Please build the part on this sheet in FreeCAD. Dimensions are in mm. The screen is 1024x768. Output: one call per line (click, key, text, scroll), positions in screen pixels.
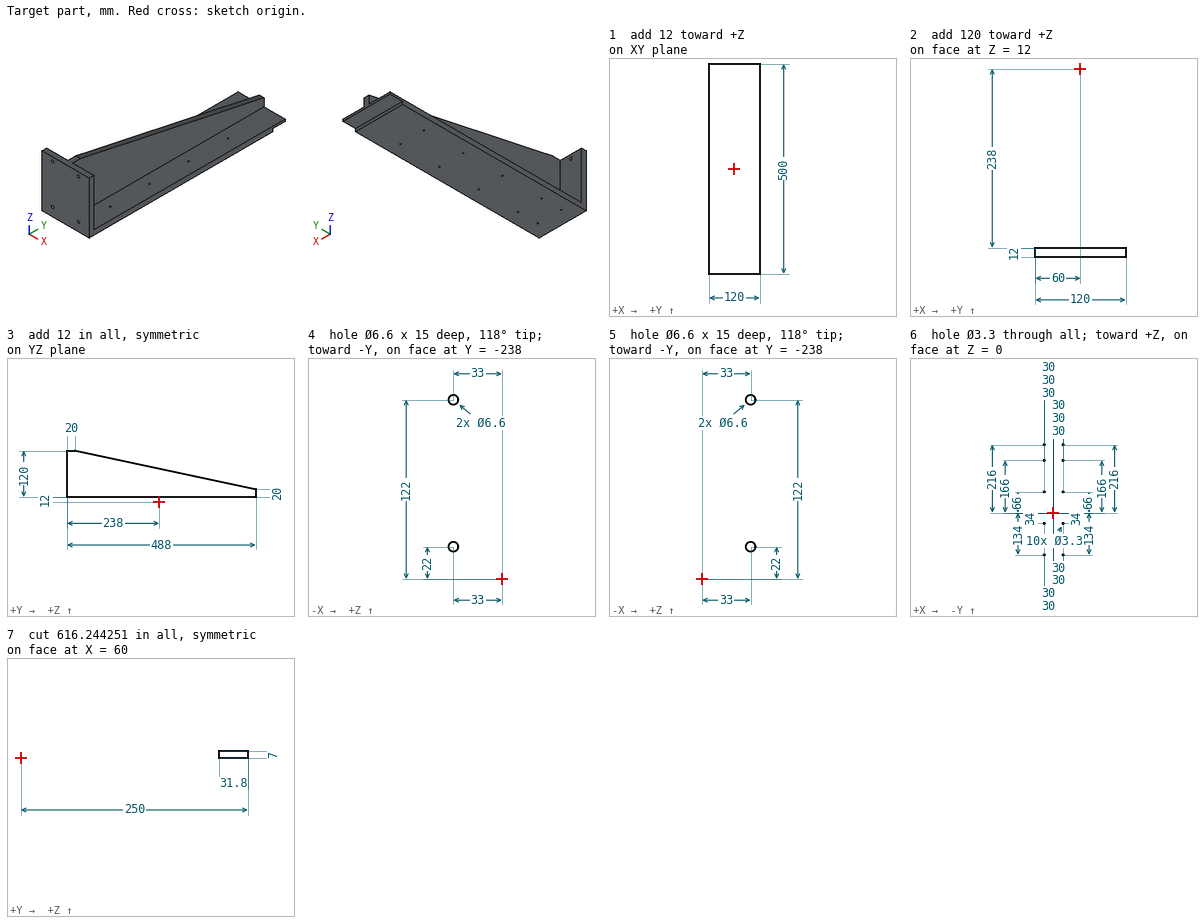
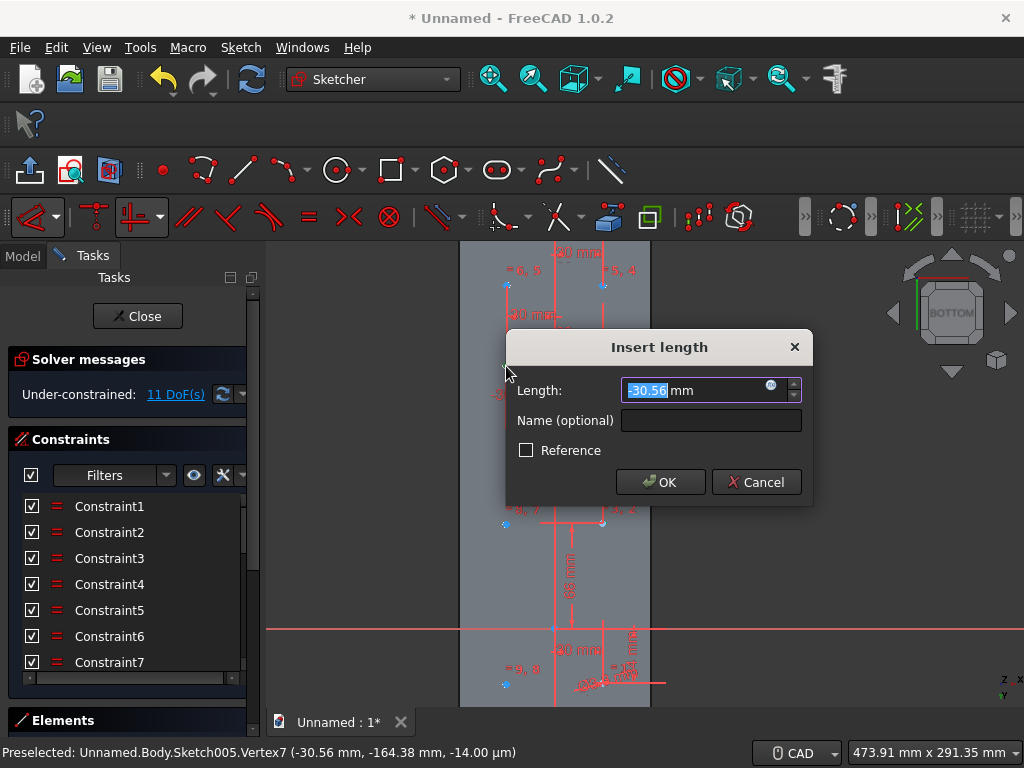
text(-30)
key(Return)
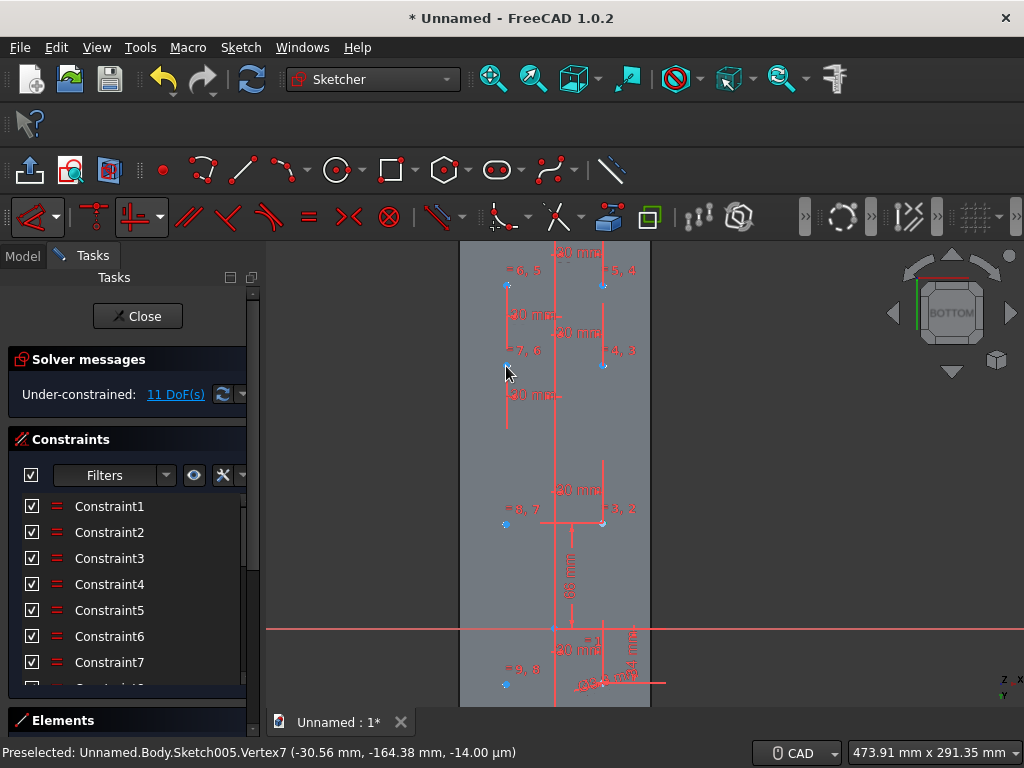
click(506, 524)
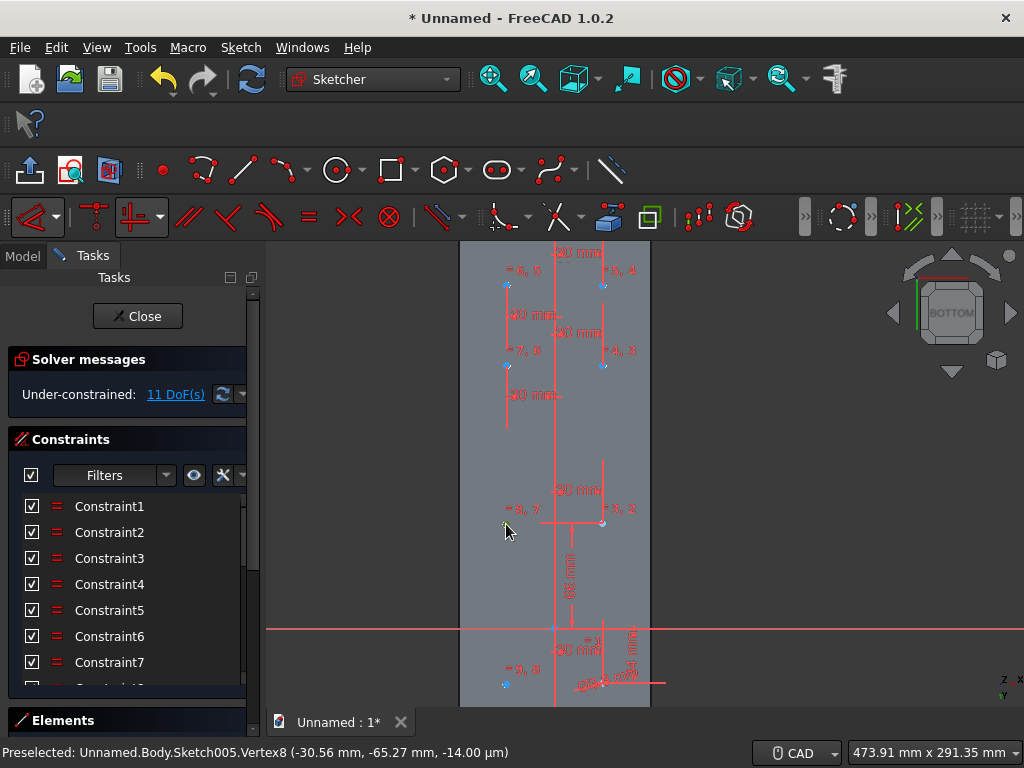
click(58, 218)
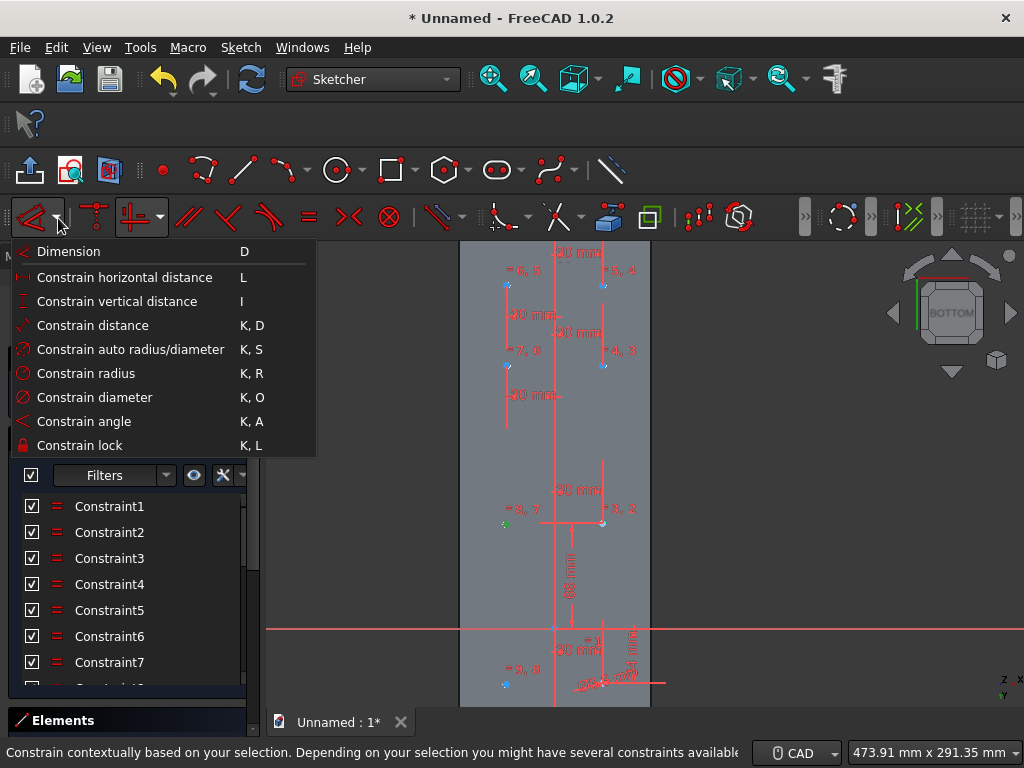
click(164, 277)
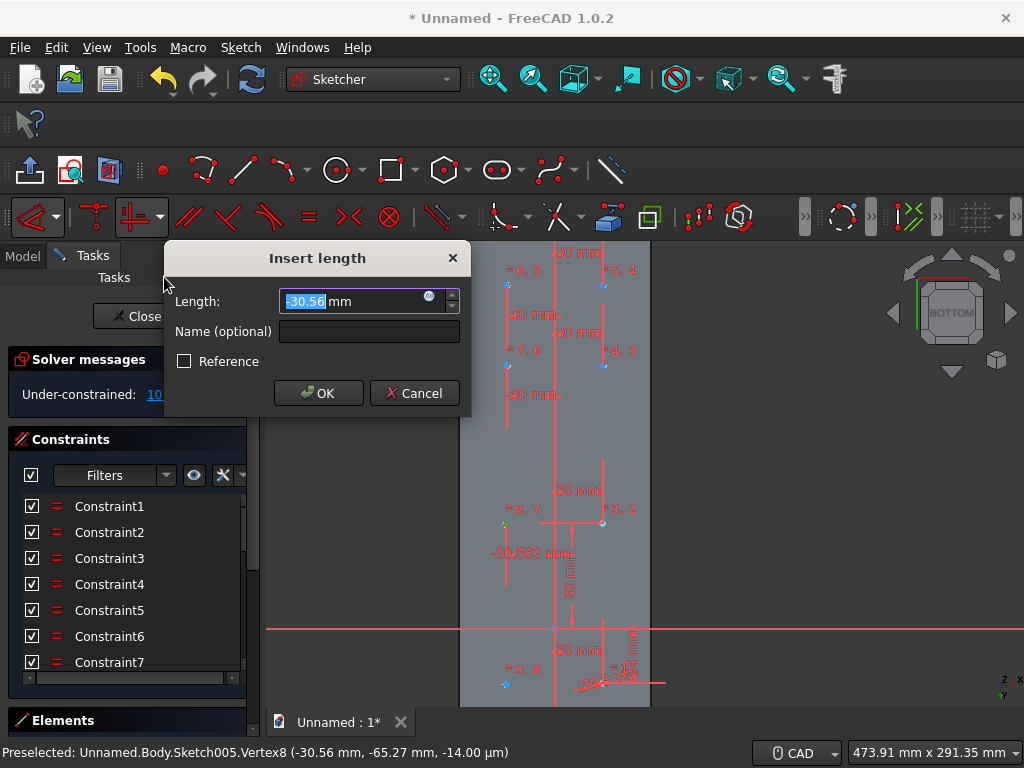
text(-30)
key(Return)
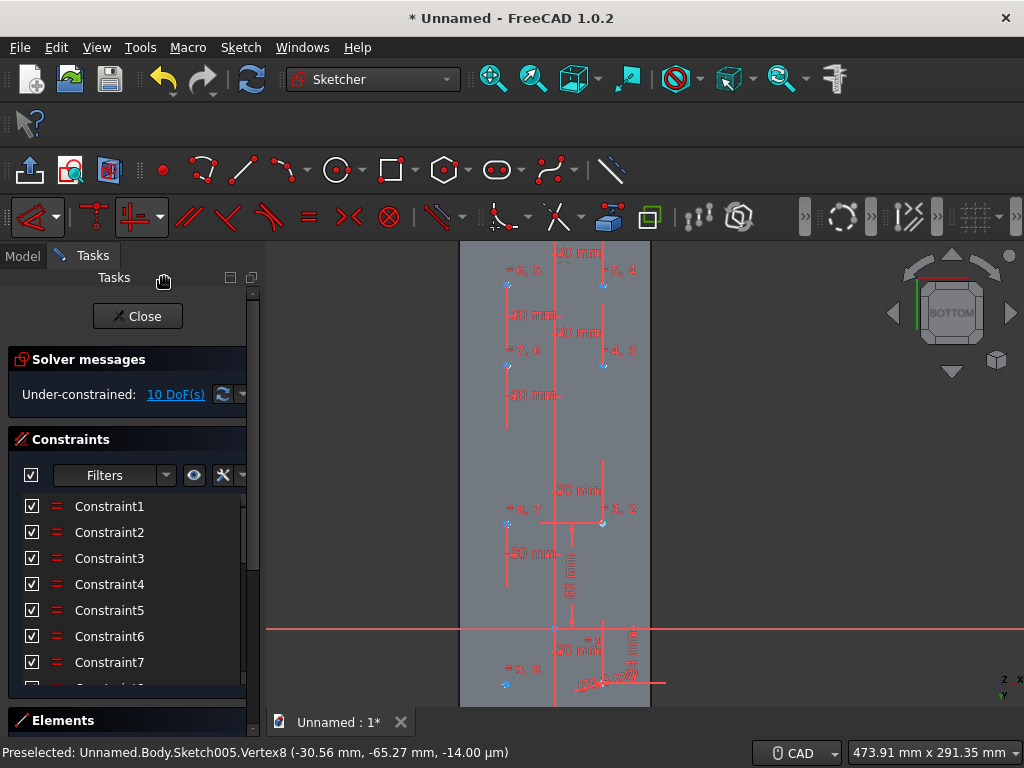
click(507, 524)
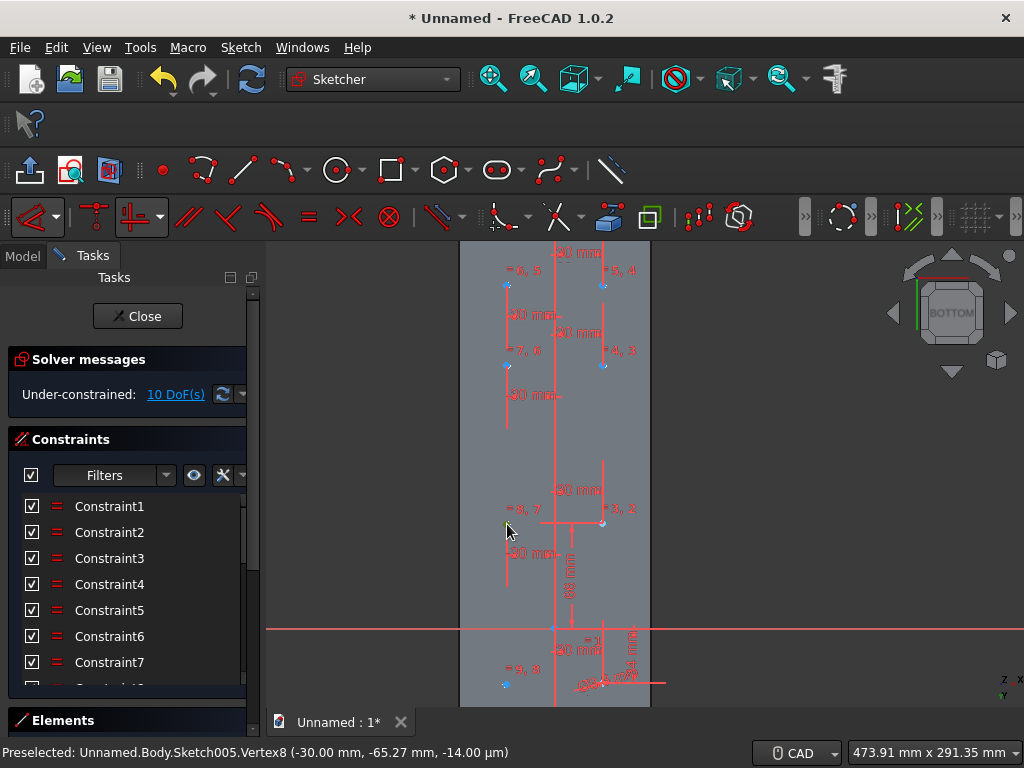
key(i)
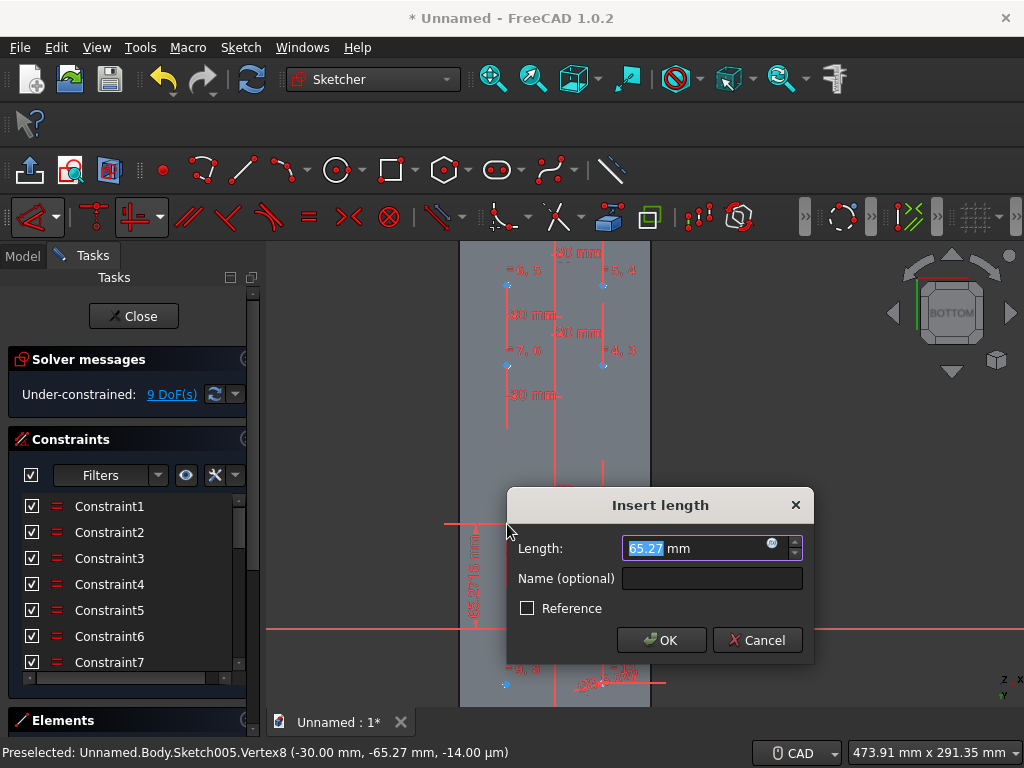
text(66)
key(Return)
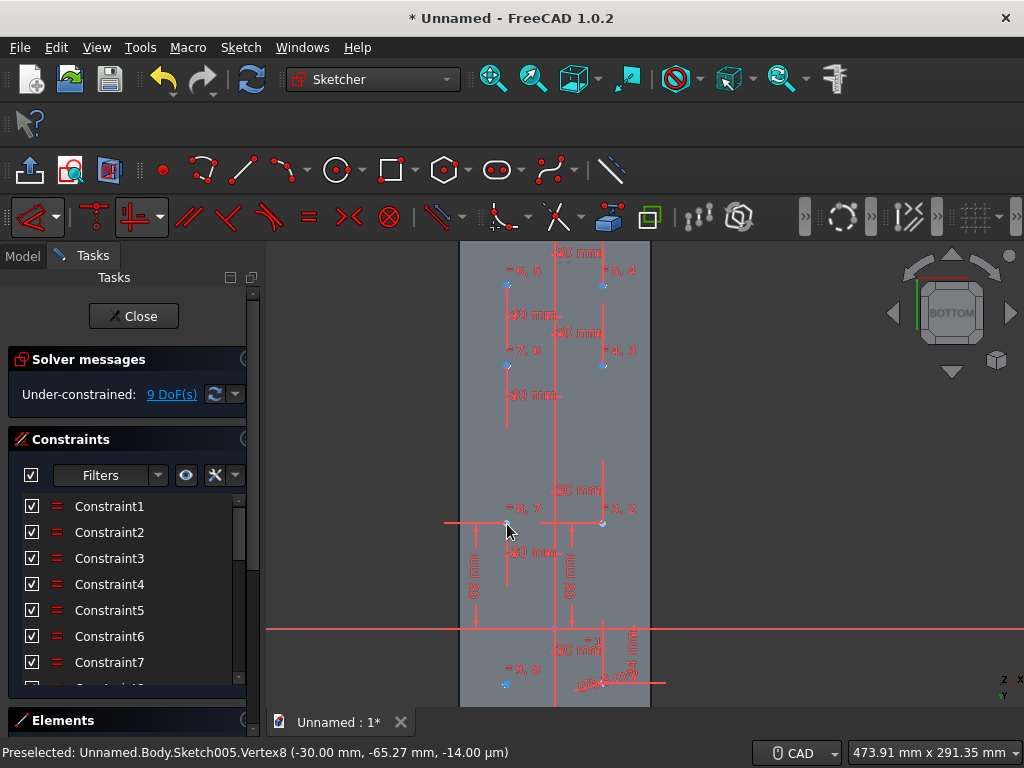
scroll(603, 366, down, 3)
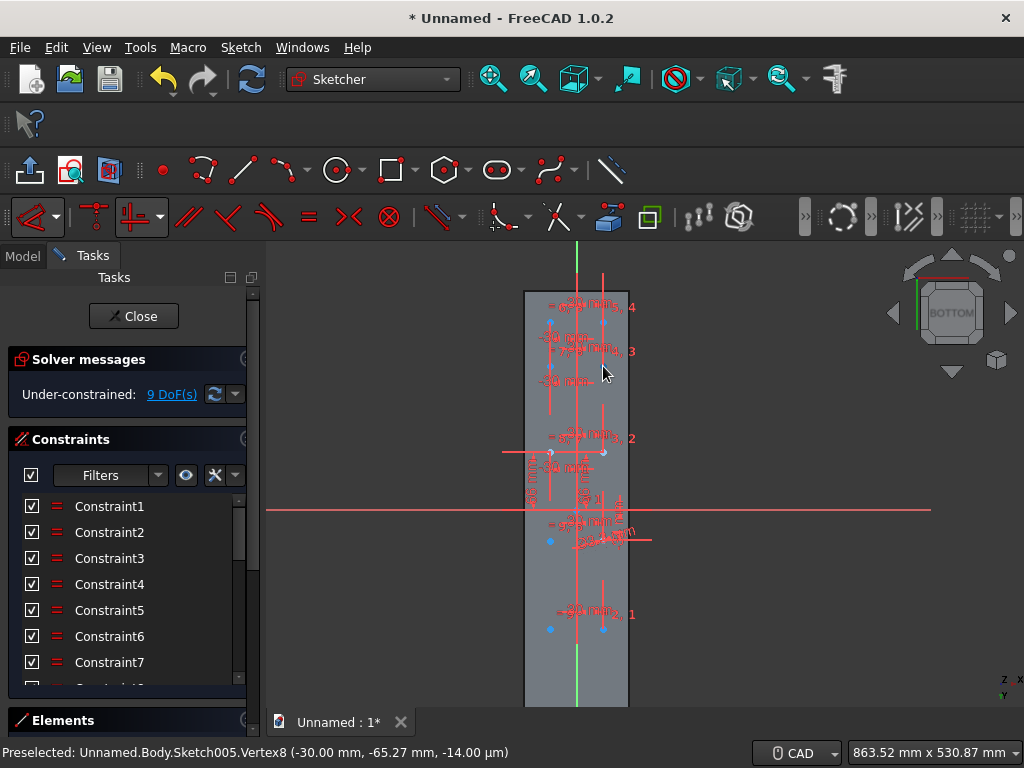
scroll(550, 541, up, 3)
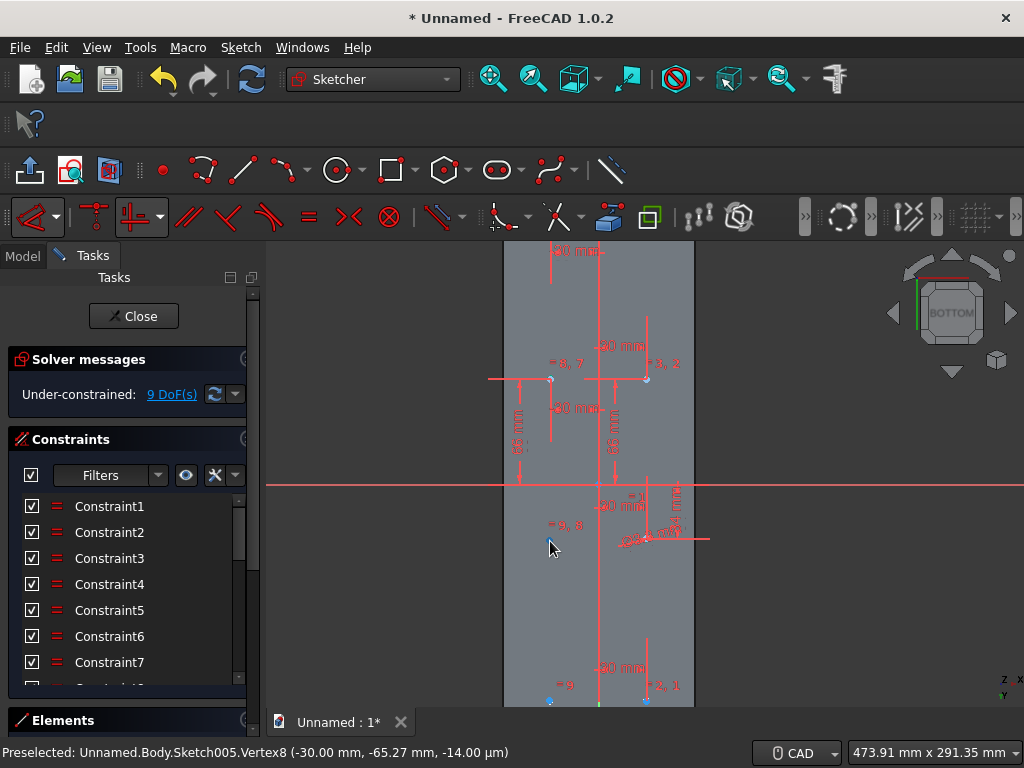
click(550, 541)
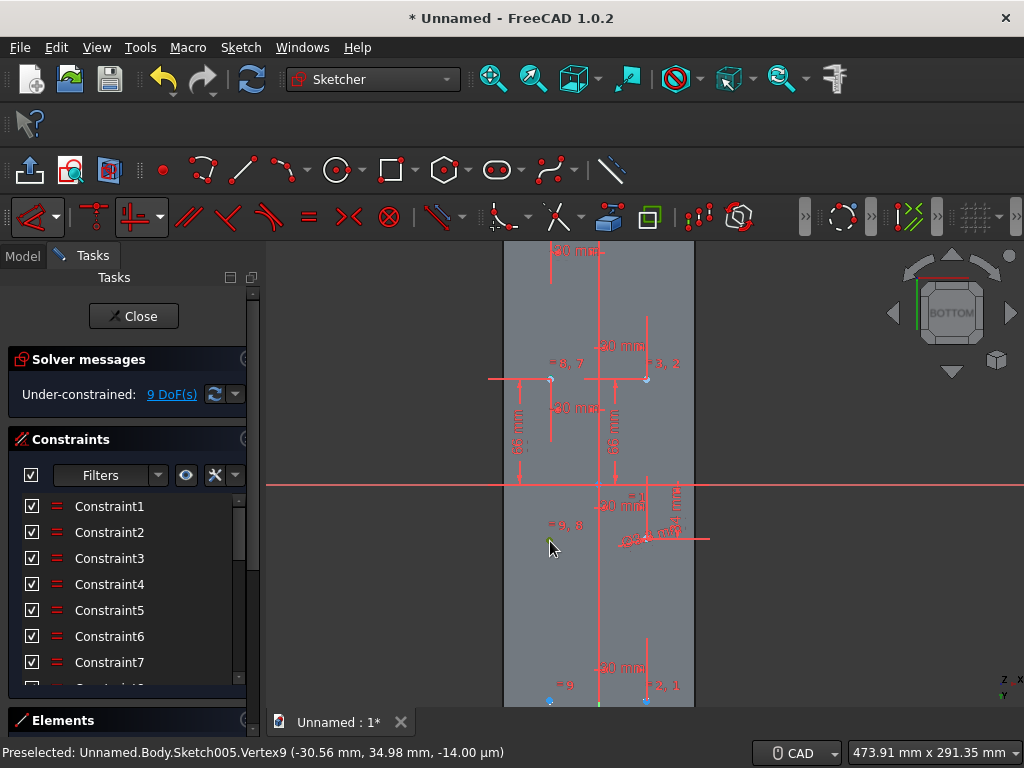
key(l)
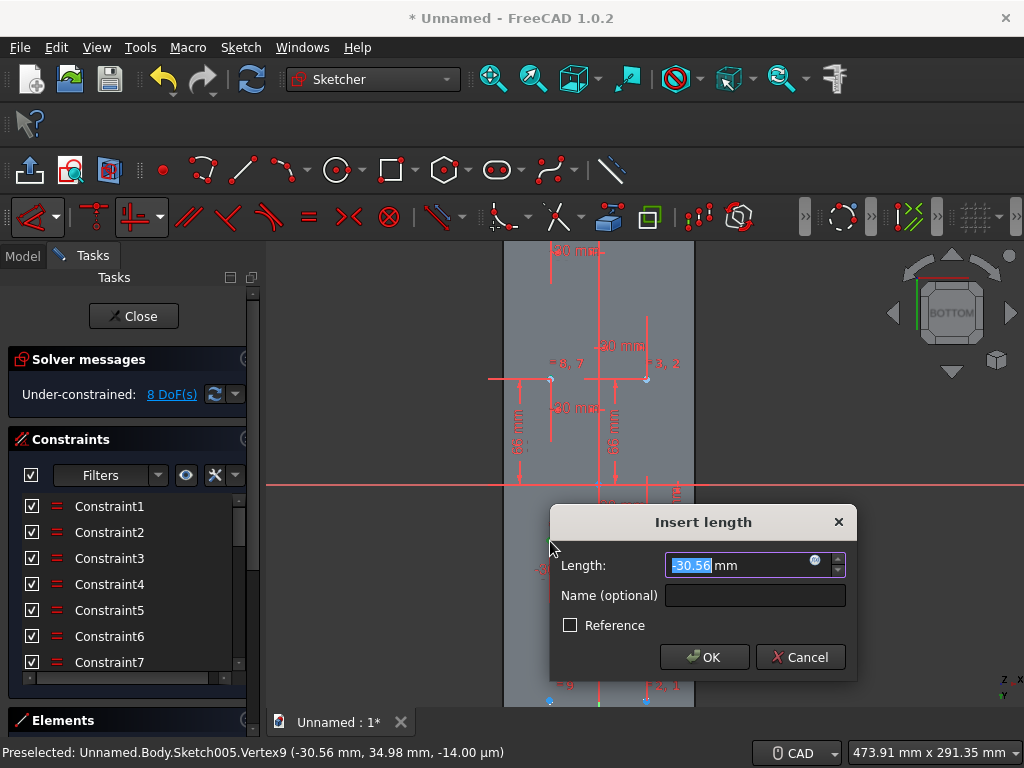
text(-30)
key(Return)